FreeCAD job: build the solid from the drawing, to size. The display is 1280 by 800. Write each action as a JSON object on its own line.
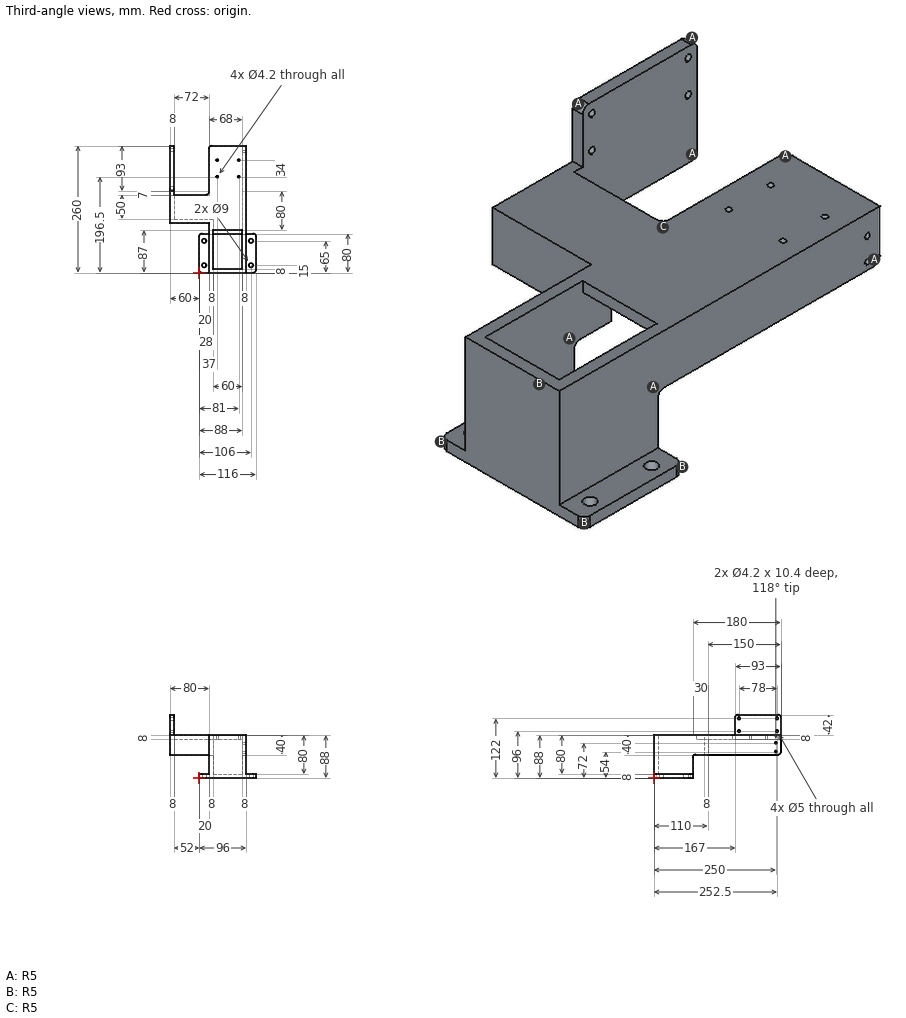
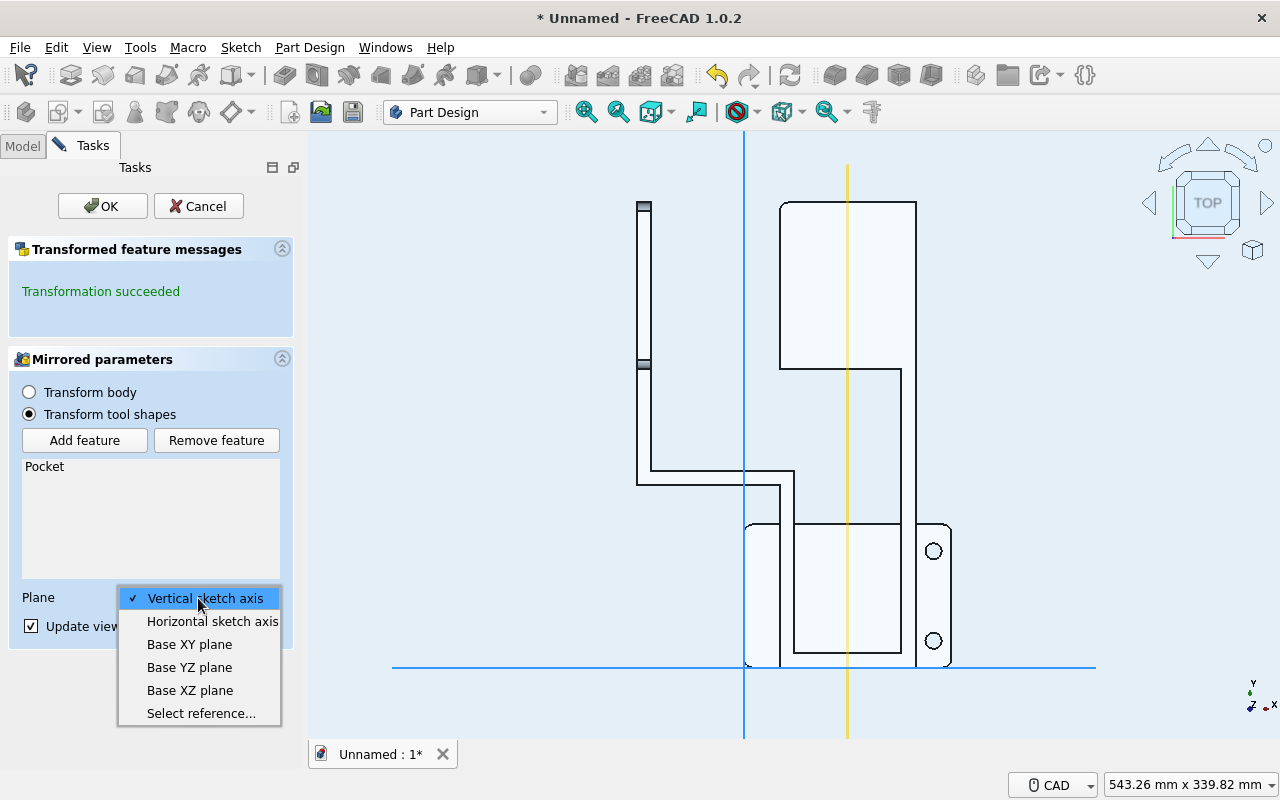
{"action": "left_click", "coordinate": [198, 714]}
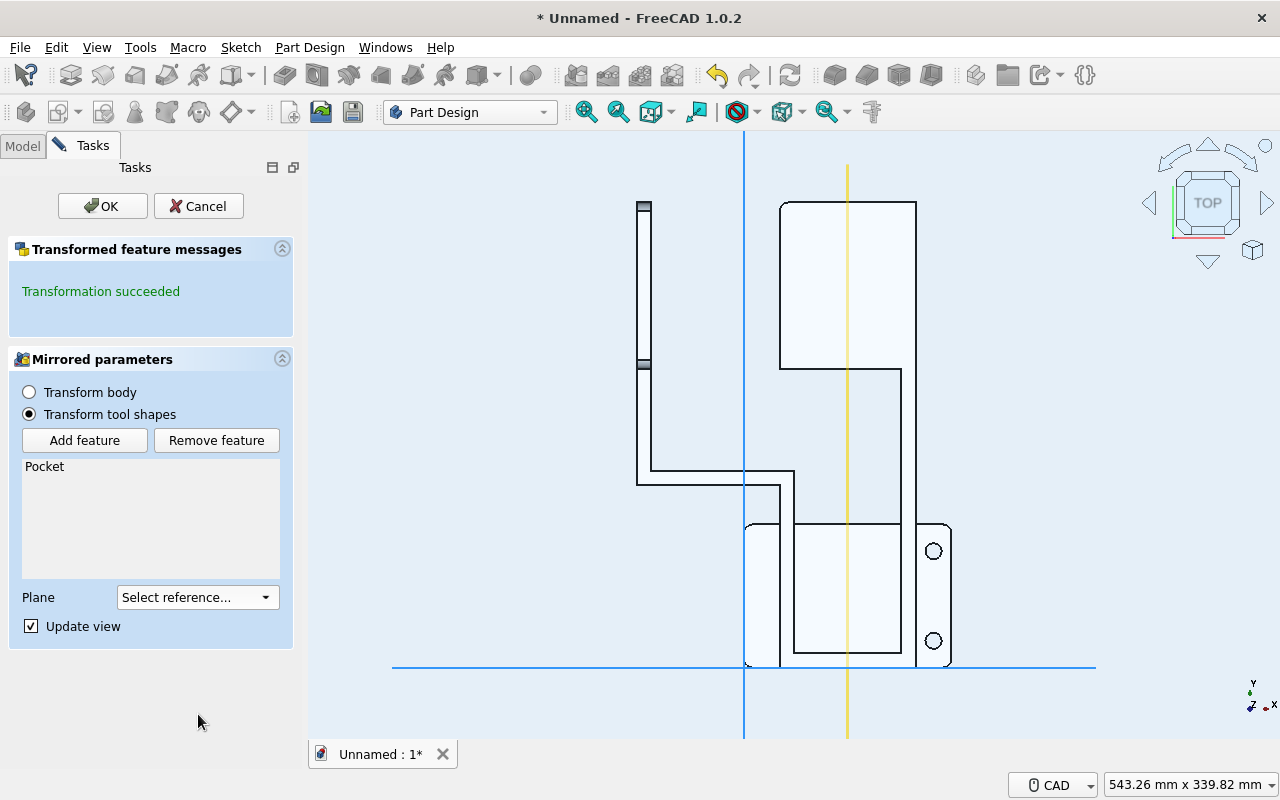
{"action": "left_click", "coordinate": [23, 145]}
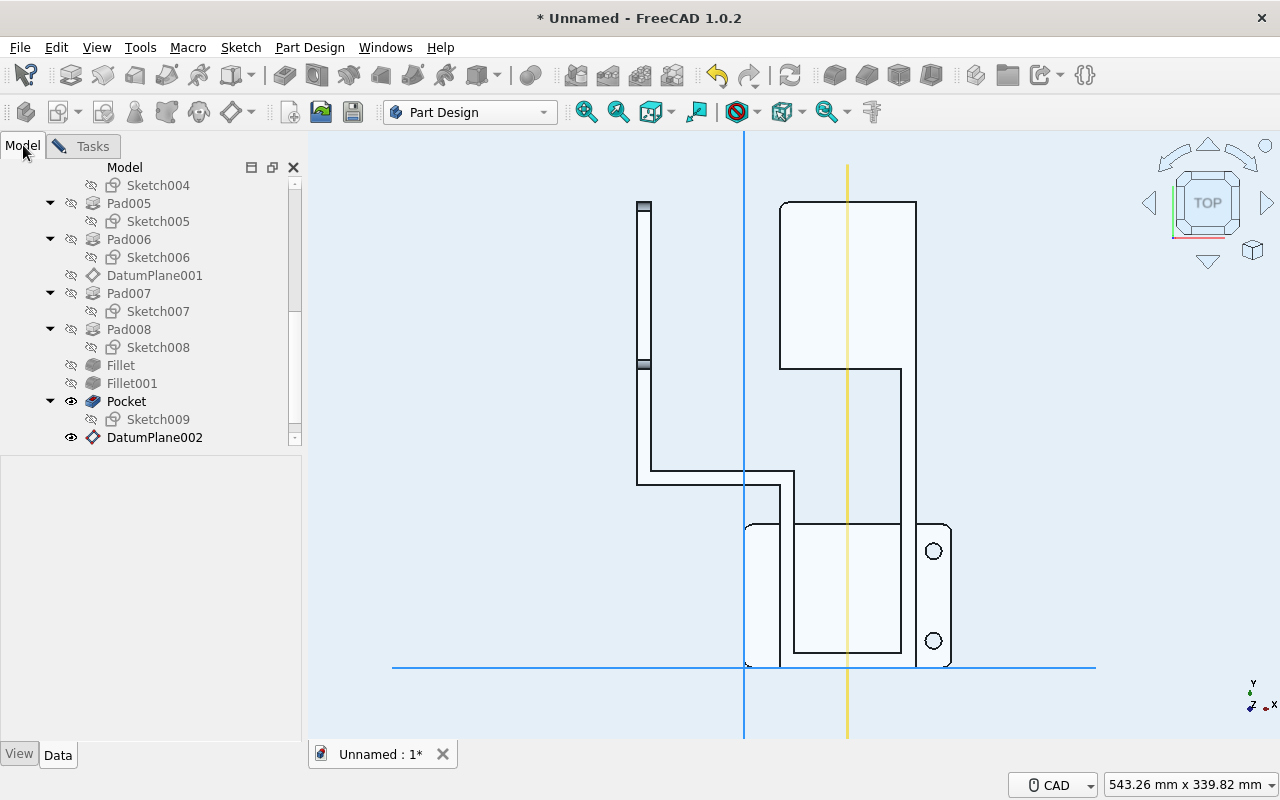
{"action": "left_click", "coordinate": [116, 437]}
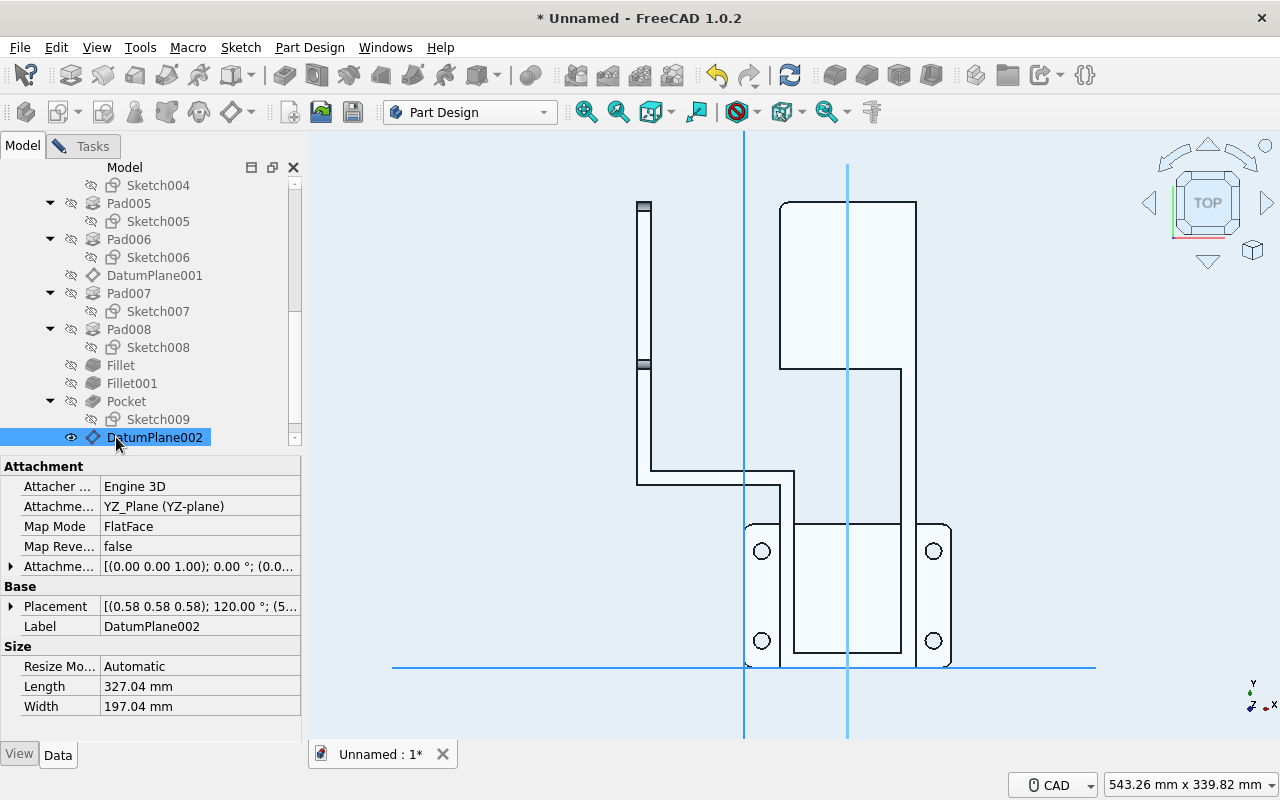
{"action": "left_click", "coordinate": [84, 145]}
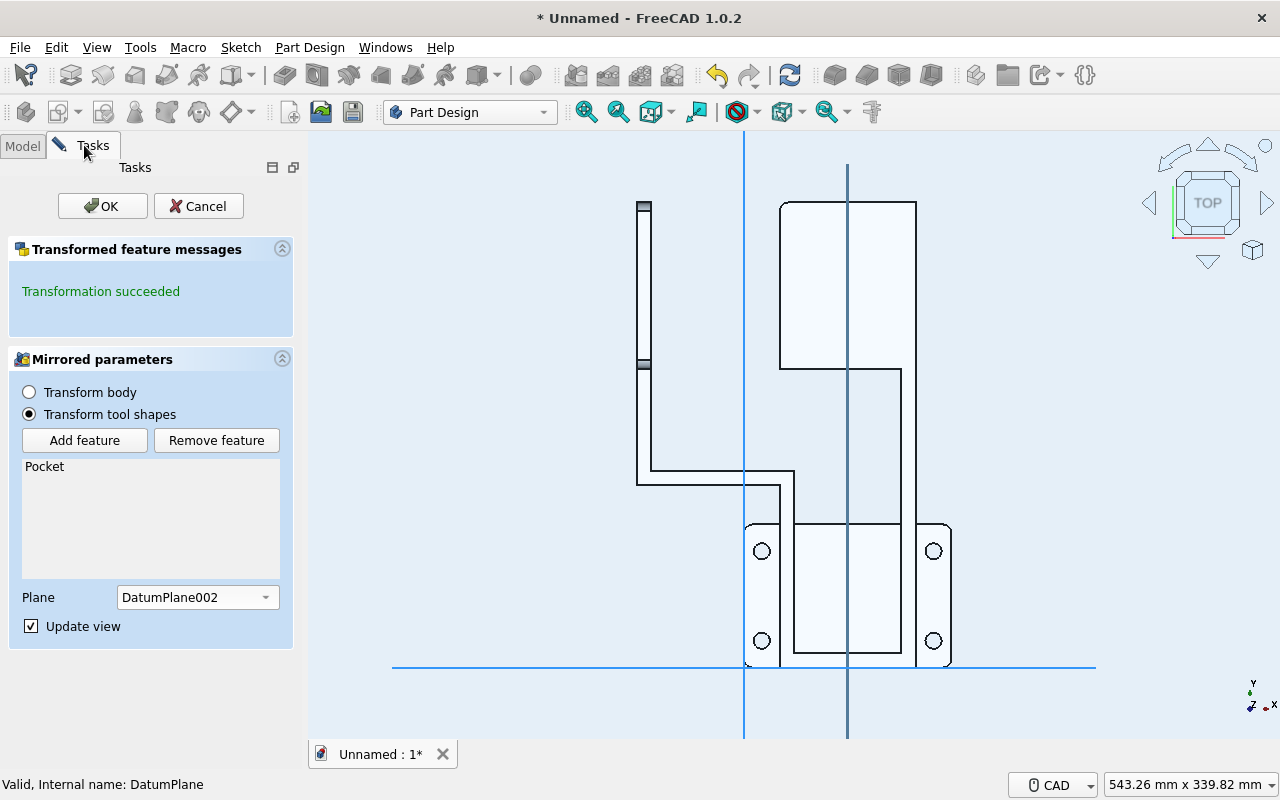
{"action": "left_click", "coordinate": [103, 206]}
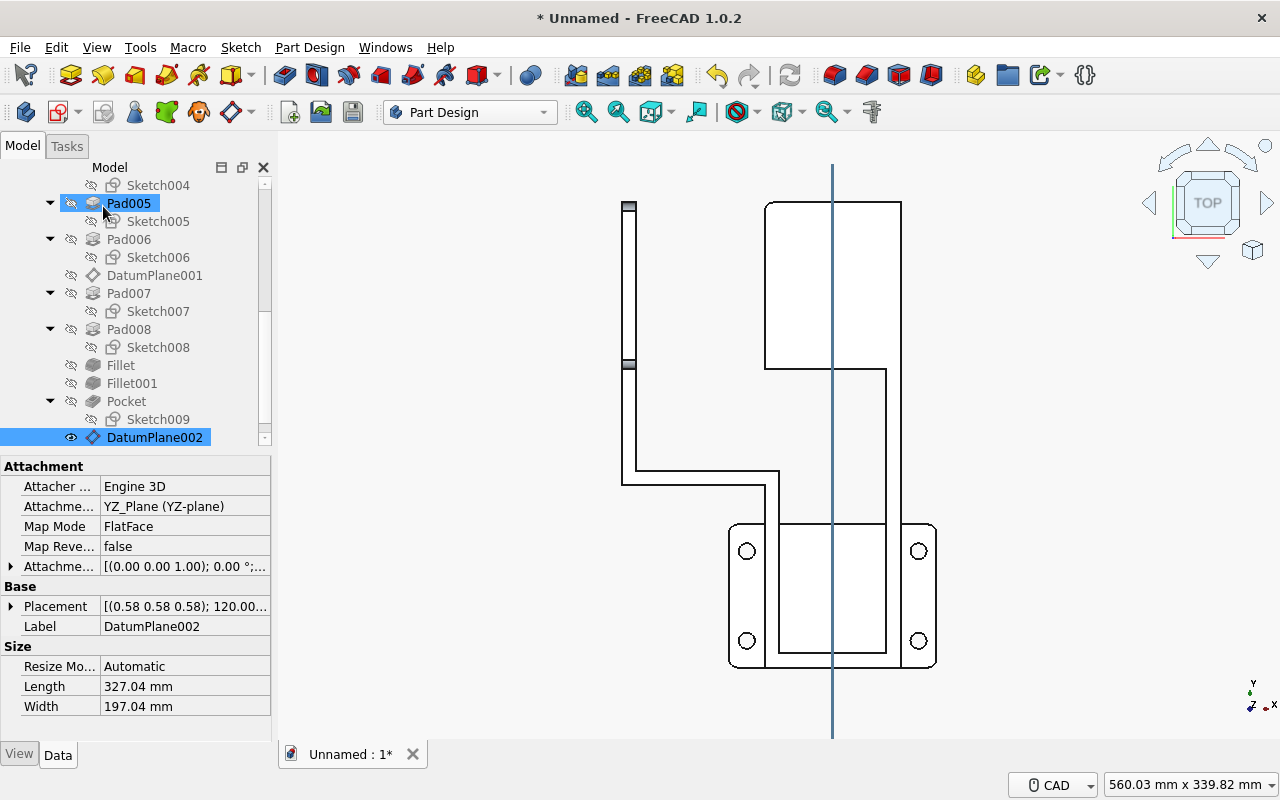
{"action": "left_click", "coordinate": [116, 437]}
{"action": "key", "text": "space"}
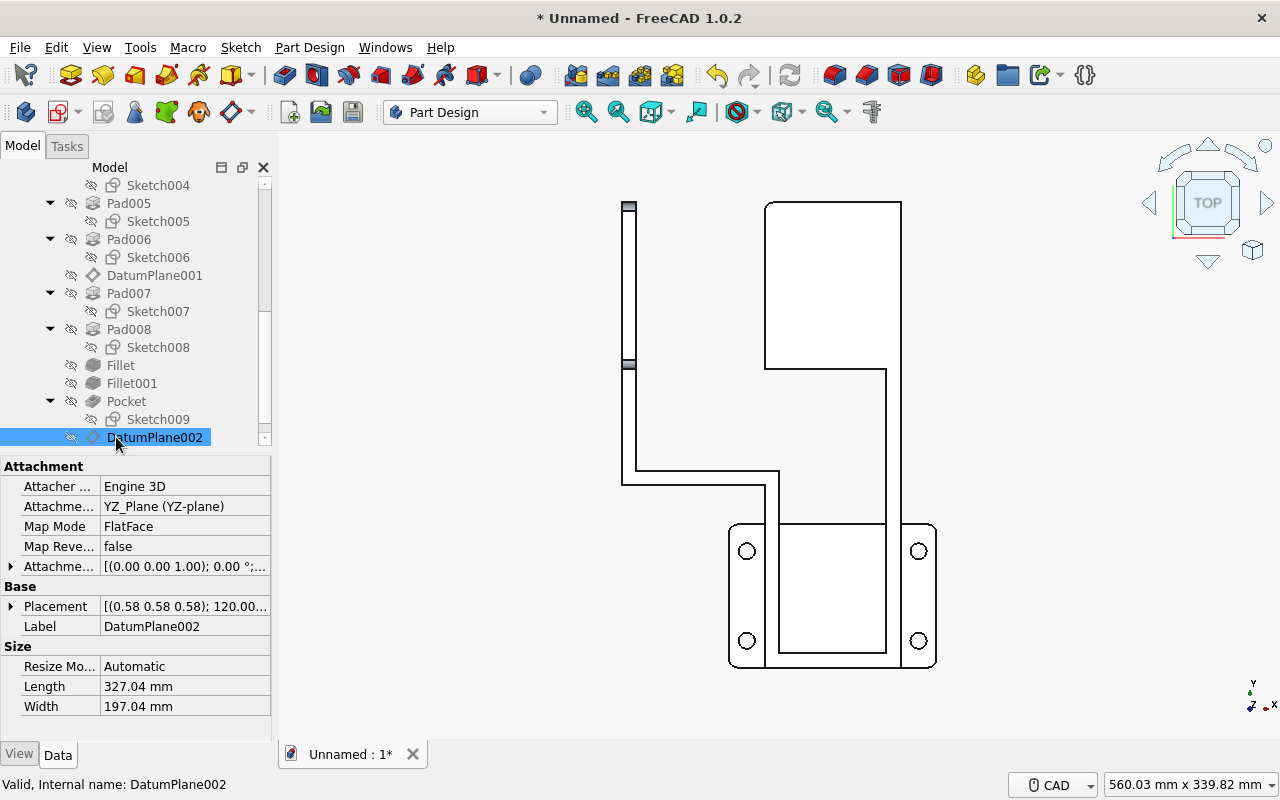
{"action": "left_click", "coordinate": [841, 301]}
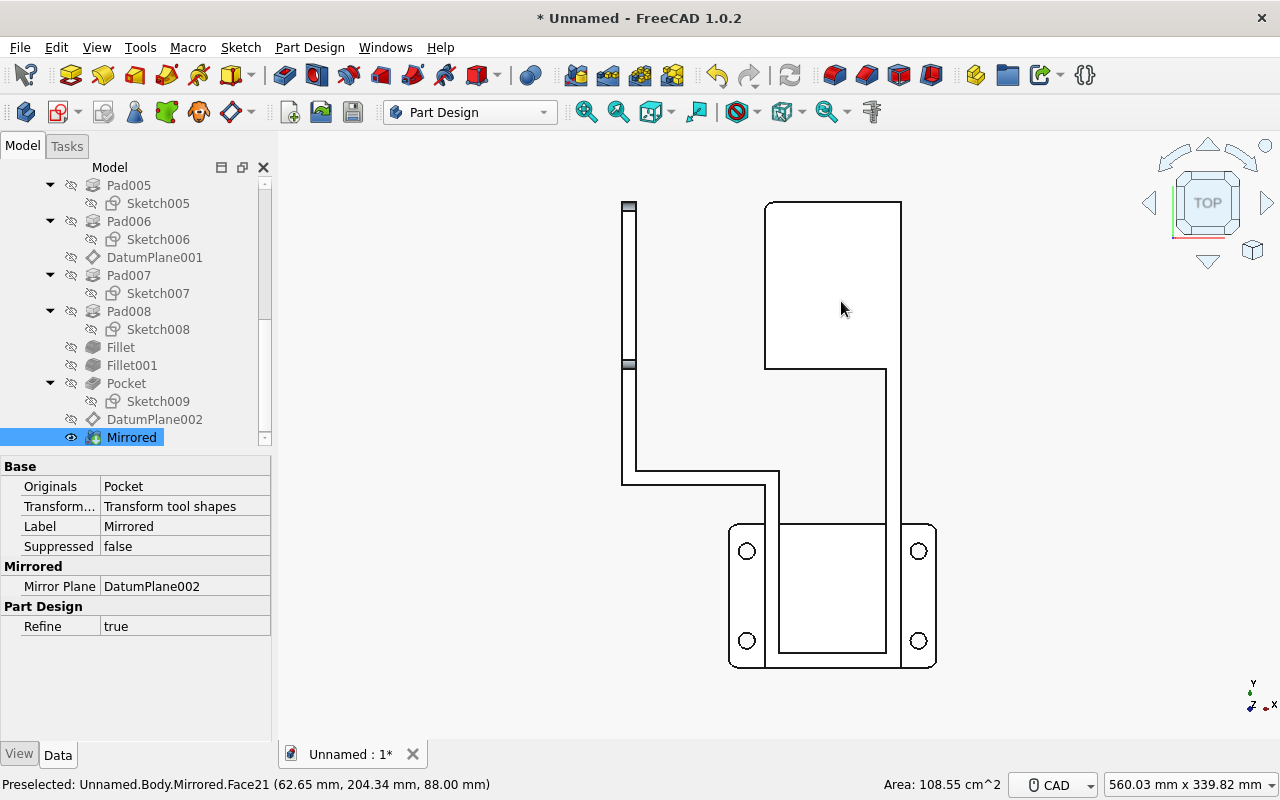
{"action": "left_click", "coordinate": [58, 112]}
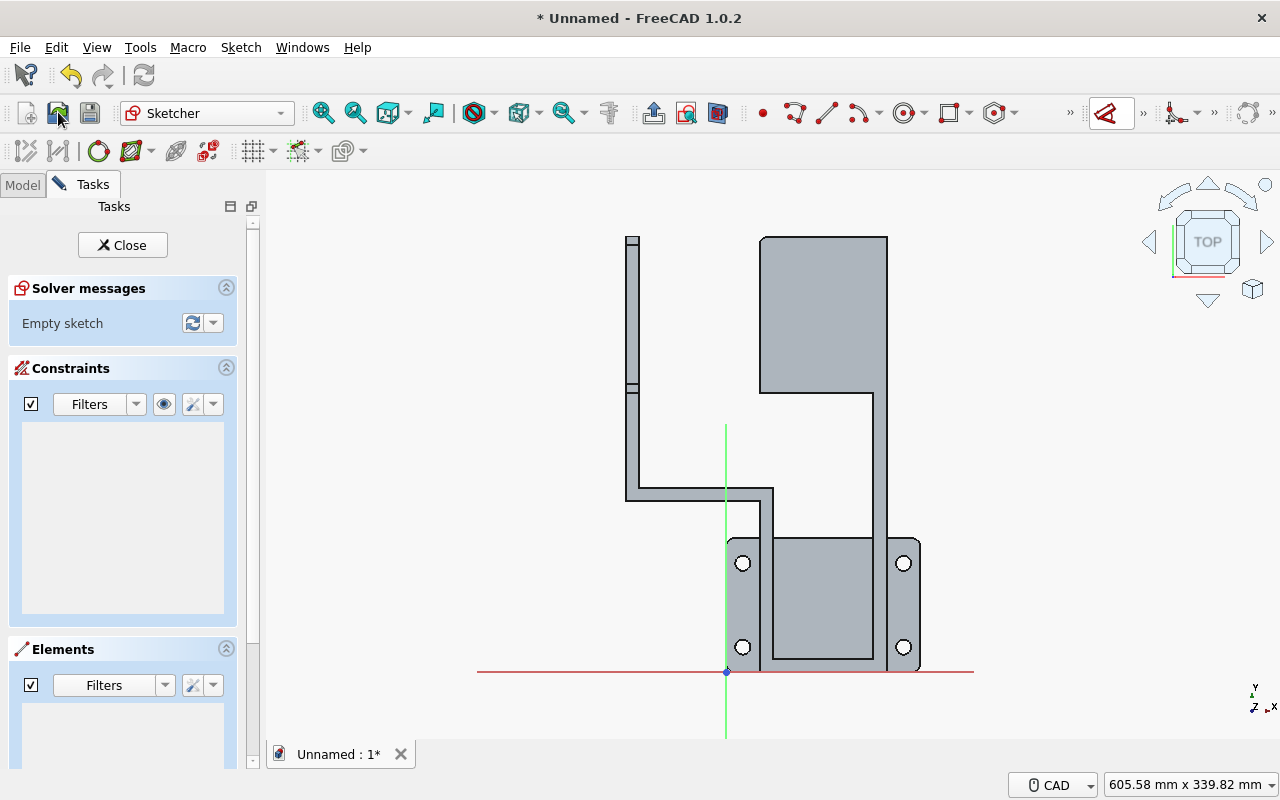
{"action": "scroll", "coordinate": [849, 287], "scroll_direction": "up", "scroll_amount": 9}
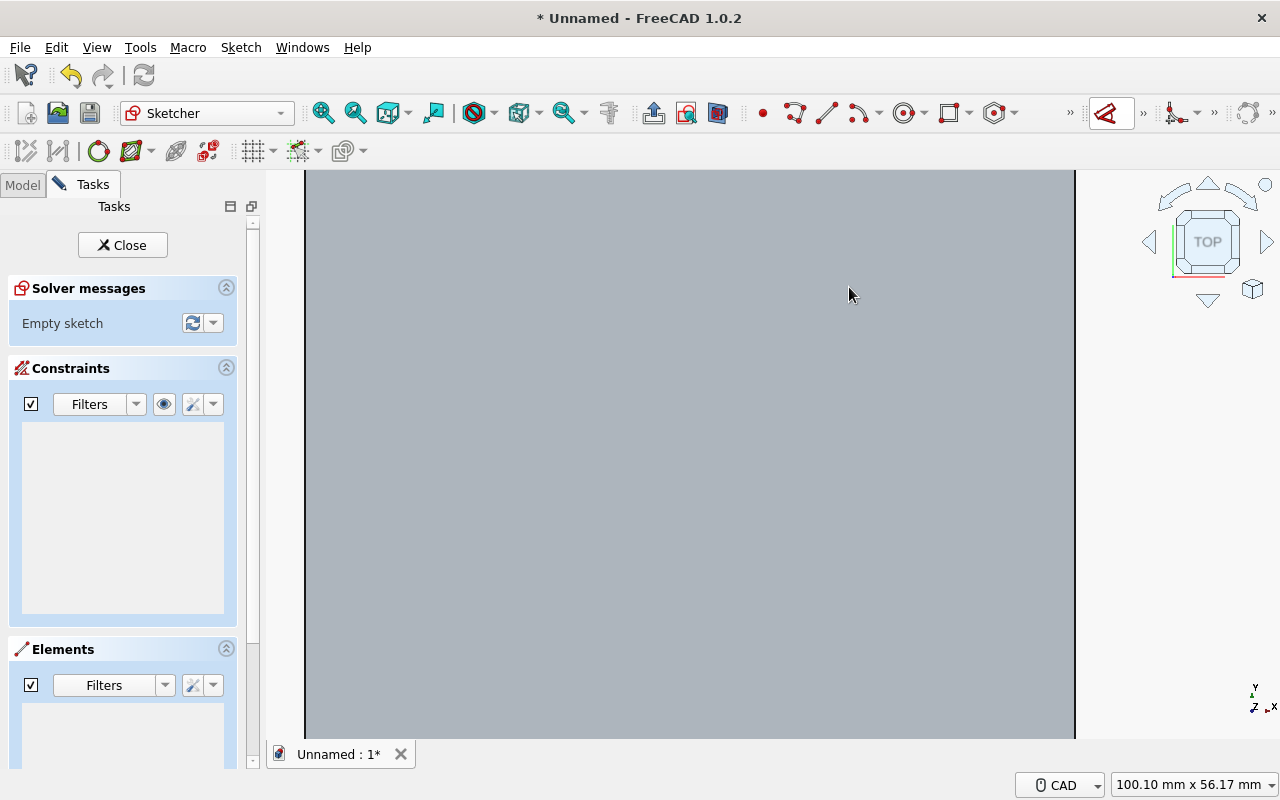
{"action": "left_click", "coordinate": [904, 114]}